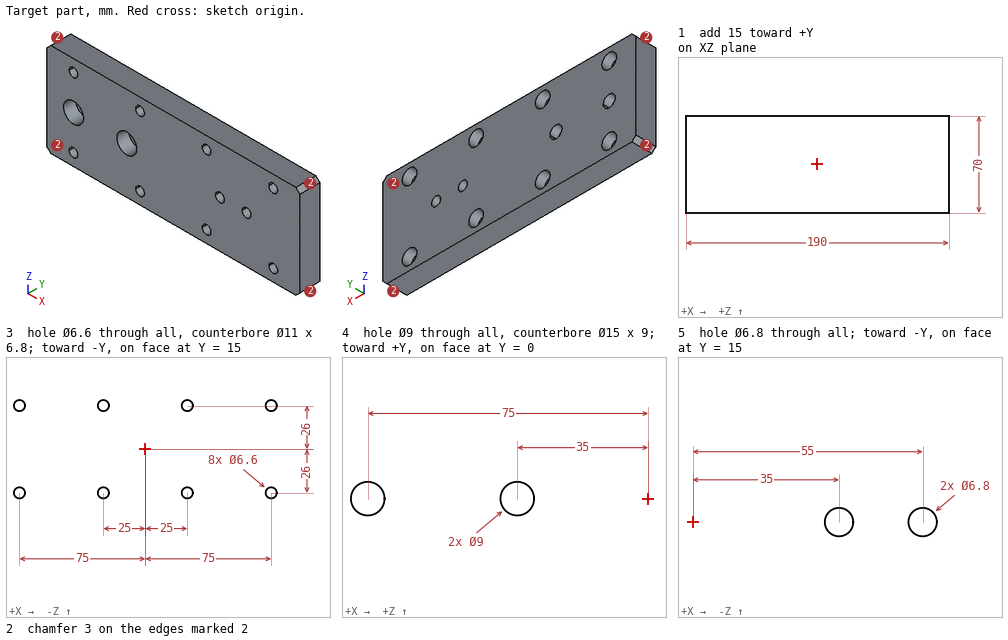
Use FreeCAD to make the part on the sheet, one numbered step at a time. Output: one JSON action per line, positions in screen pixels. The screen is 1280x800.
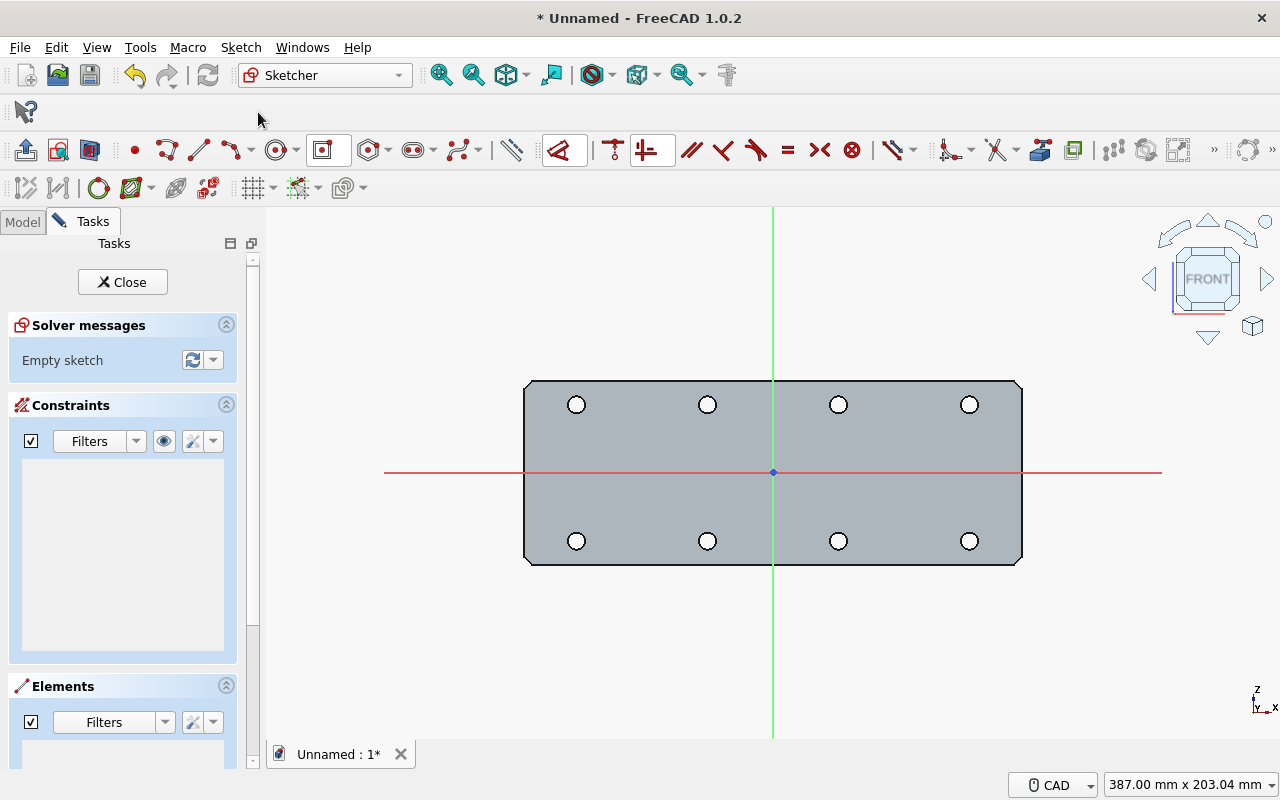
{"action": "scroll", "coordinate": [648, 473], "scroll_direction": "up", "scroll_amount": 5}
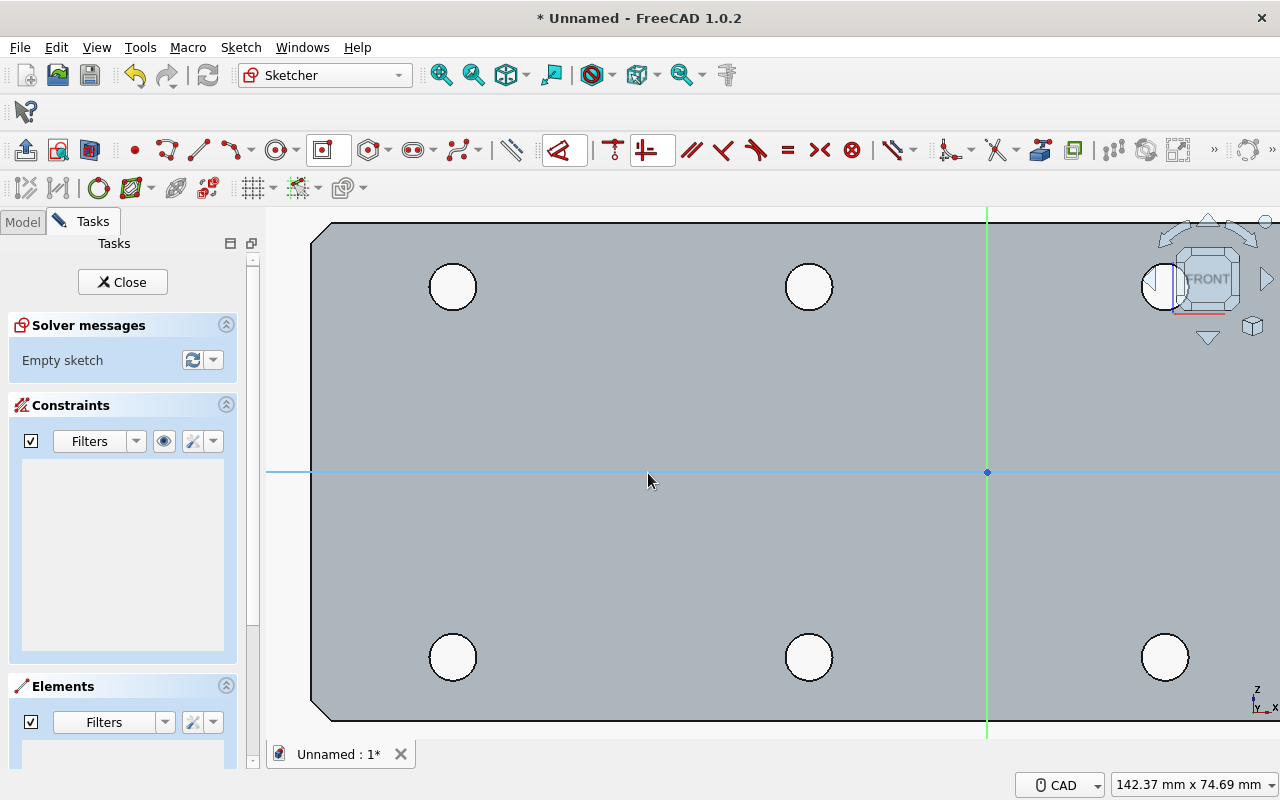
{"action": "left_click", "coordinate": [276, 150]}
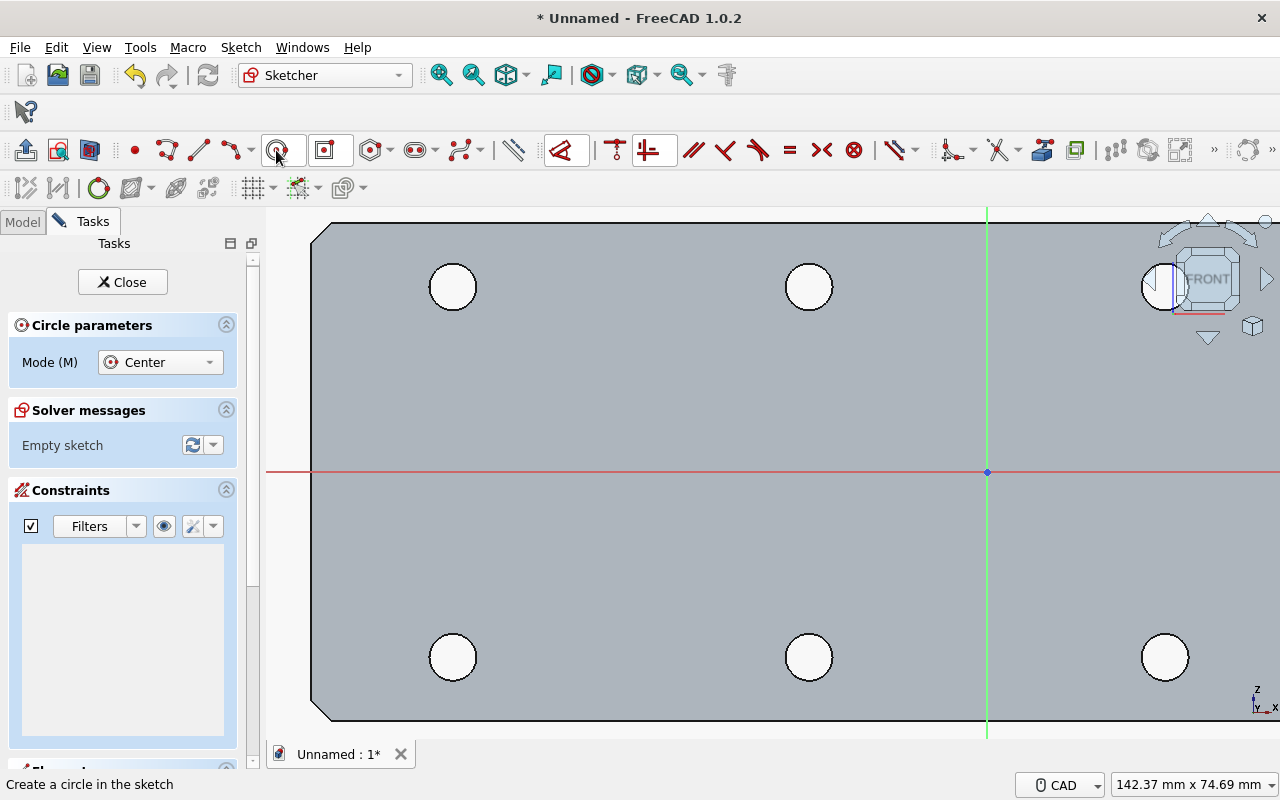
{"action": "left_click", "coordinate": [738, 472]}
{"action": "mouse_move", "coordinate": [761, 449]}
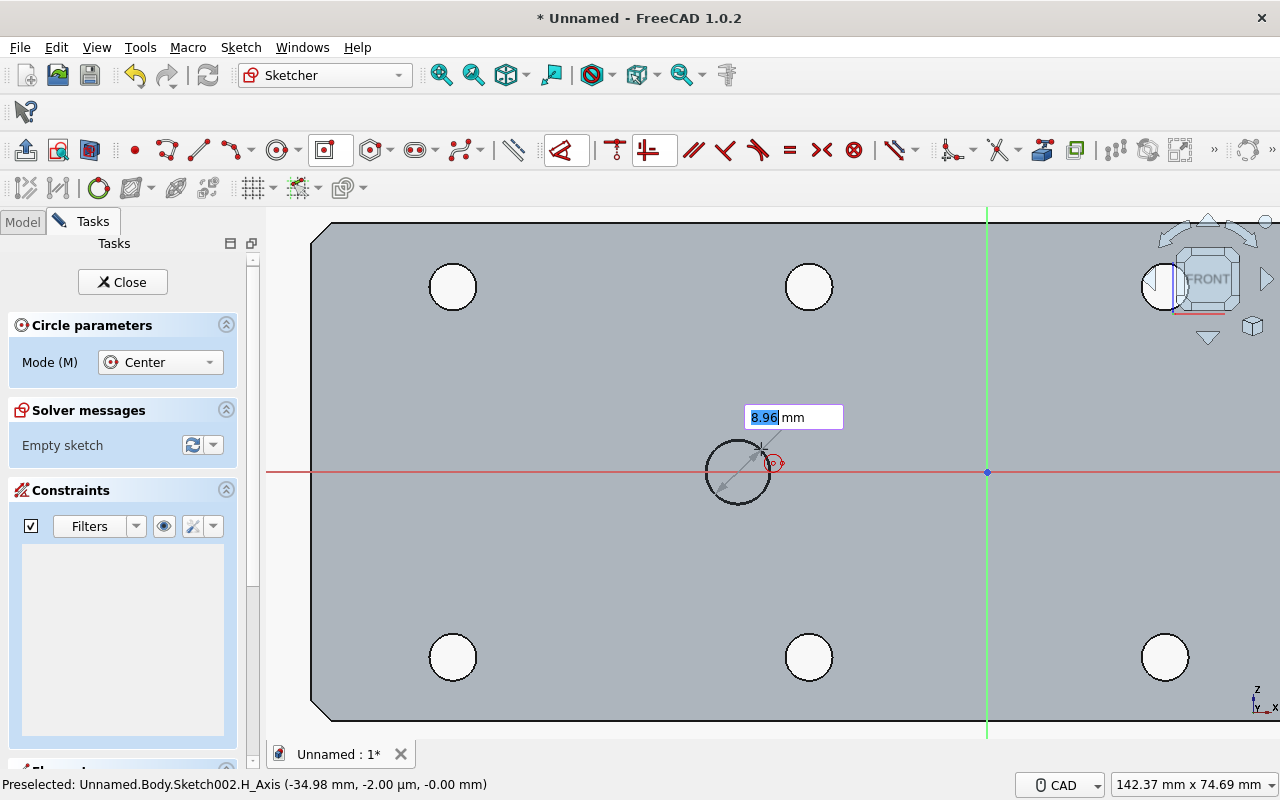
{"action": "type", "text": "9"}
{"action": "key", "text": "Return"}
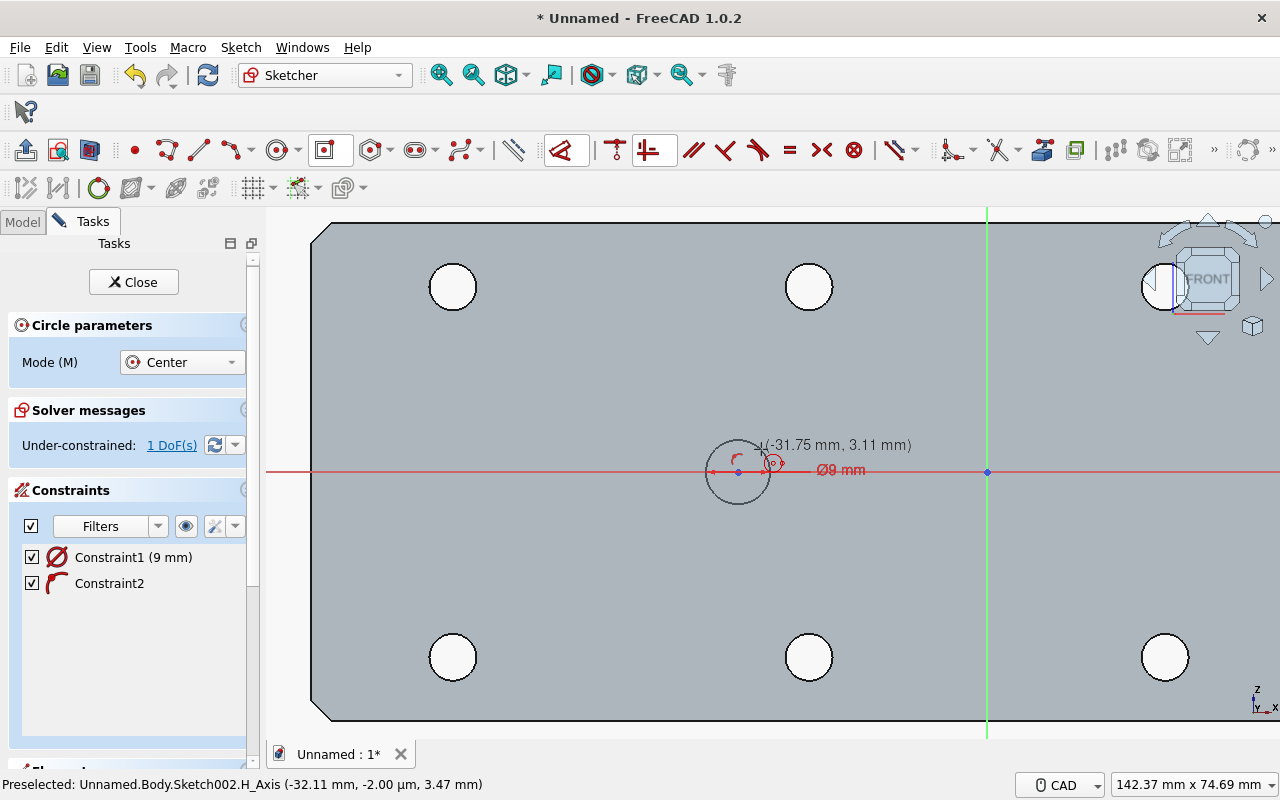
{"action": "left_click", "coordinate": [453, 472]}
{"action": "mouse_move", "coordinate": [476, 449]}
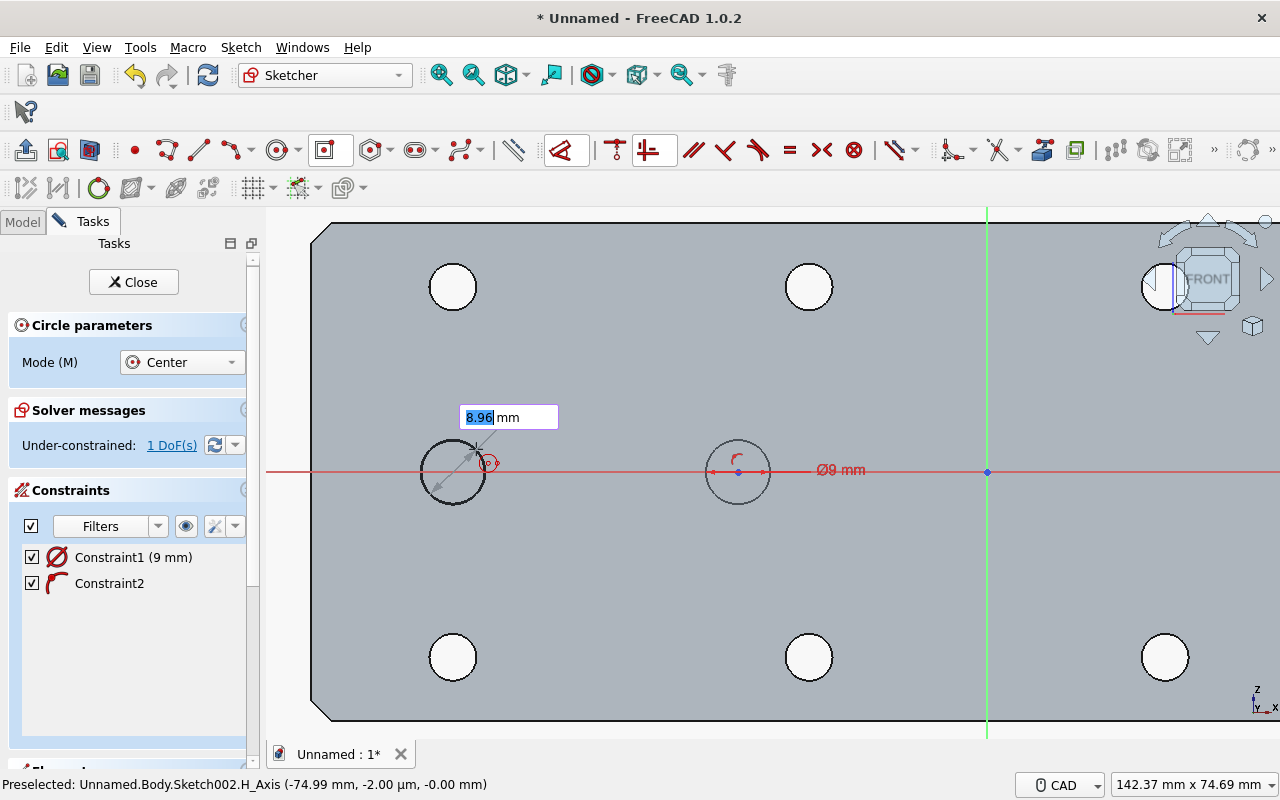
{"action": "type", "text": "9"}
{"action": "key", "text": "Return"}
{"action": "key", "text": "Escape"}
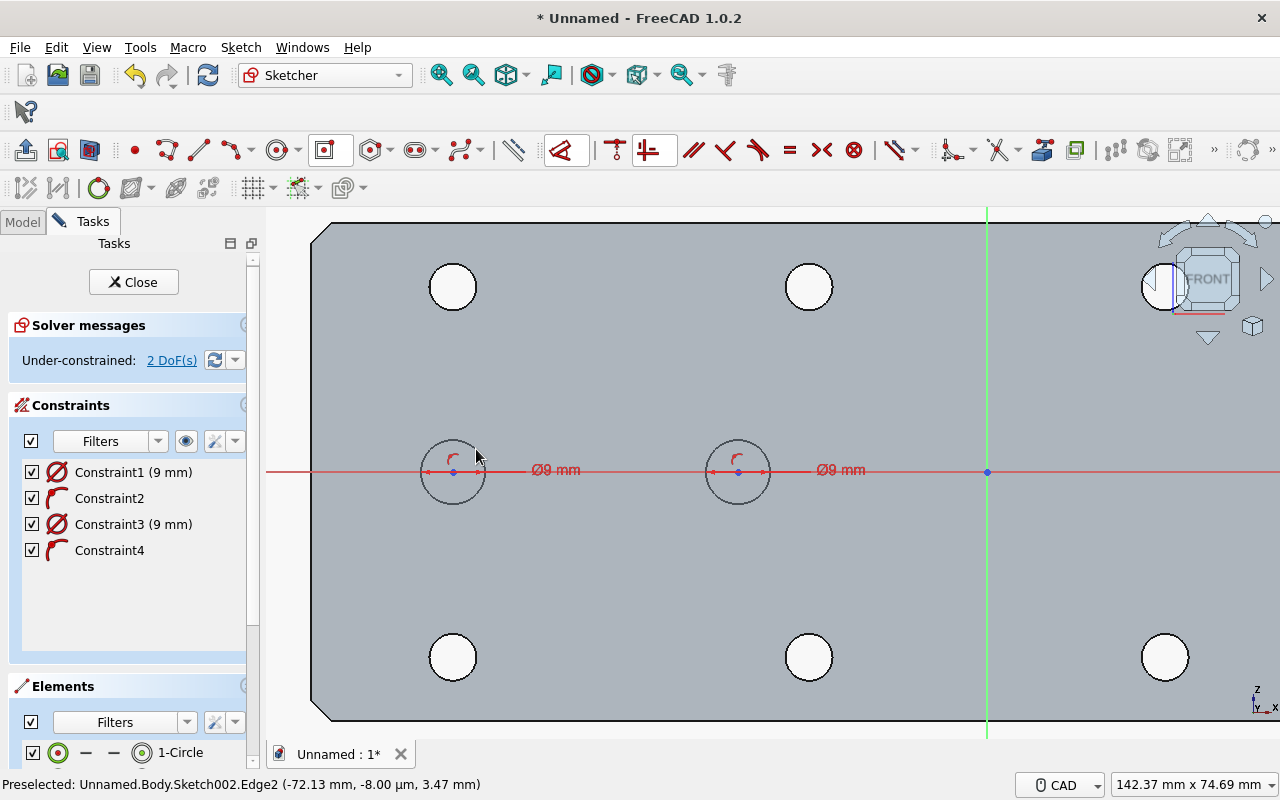
{"action": "key", "text": "d"}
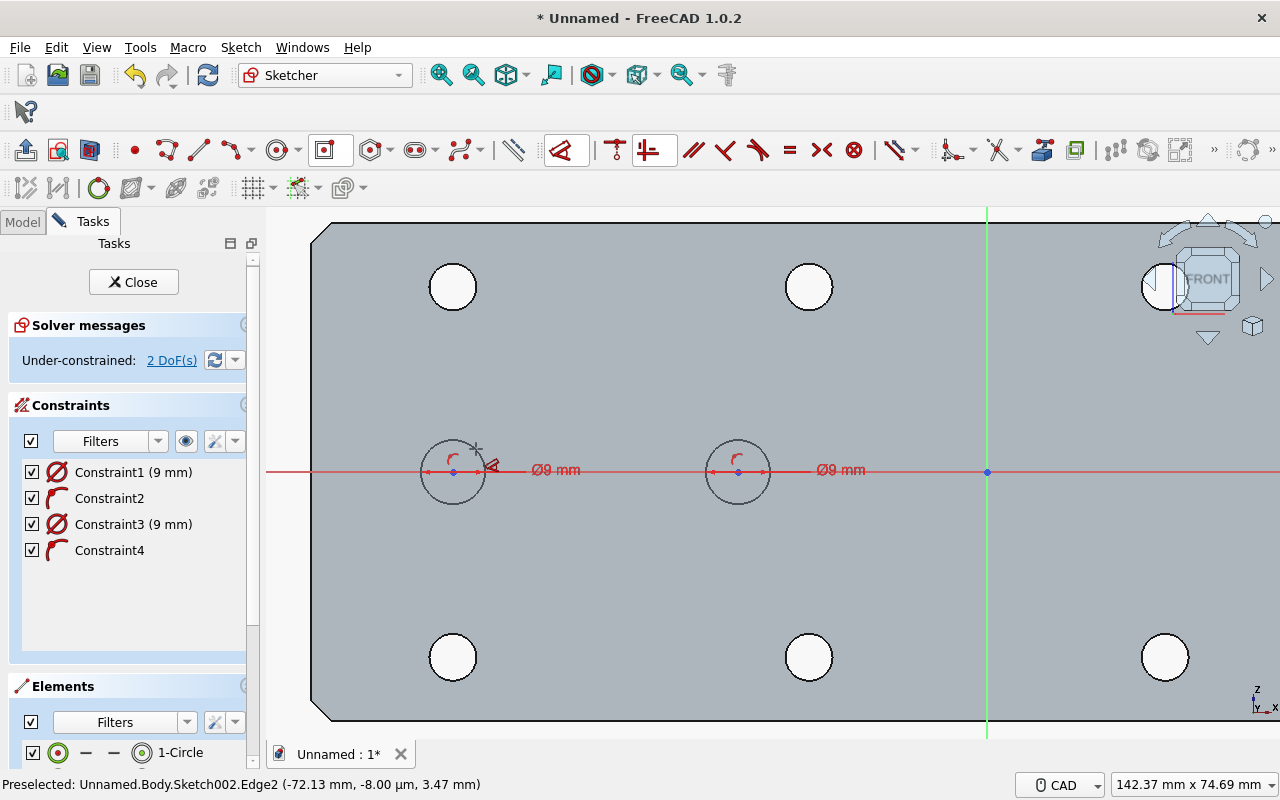
{"action": "left_click", "coordinate": [738, 472]}
{"action": "left_click", "coordinate": [863, 506]}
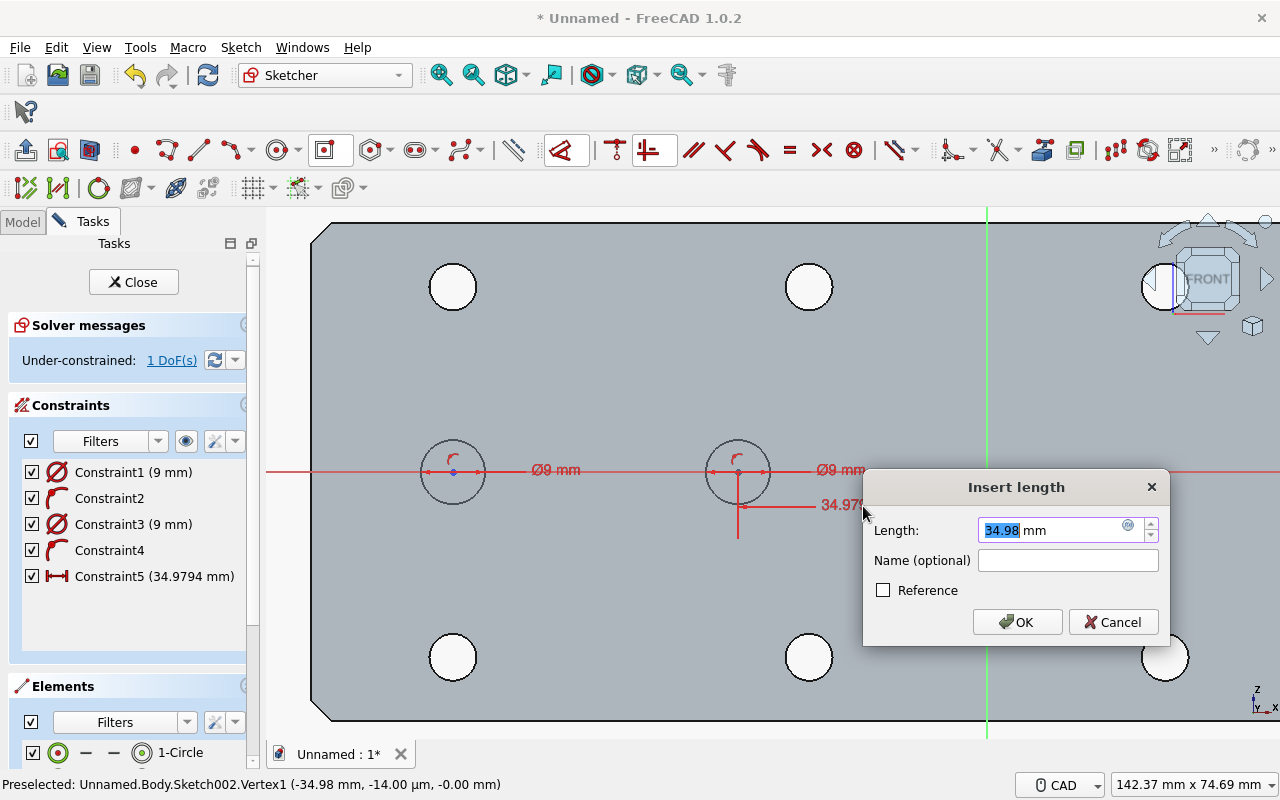
{"action": "type", "text": "35"}
{"action": "key", "text": "Return"}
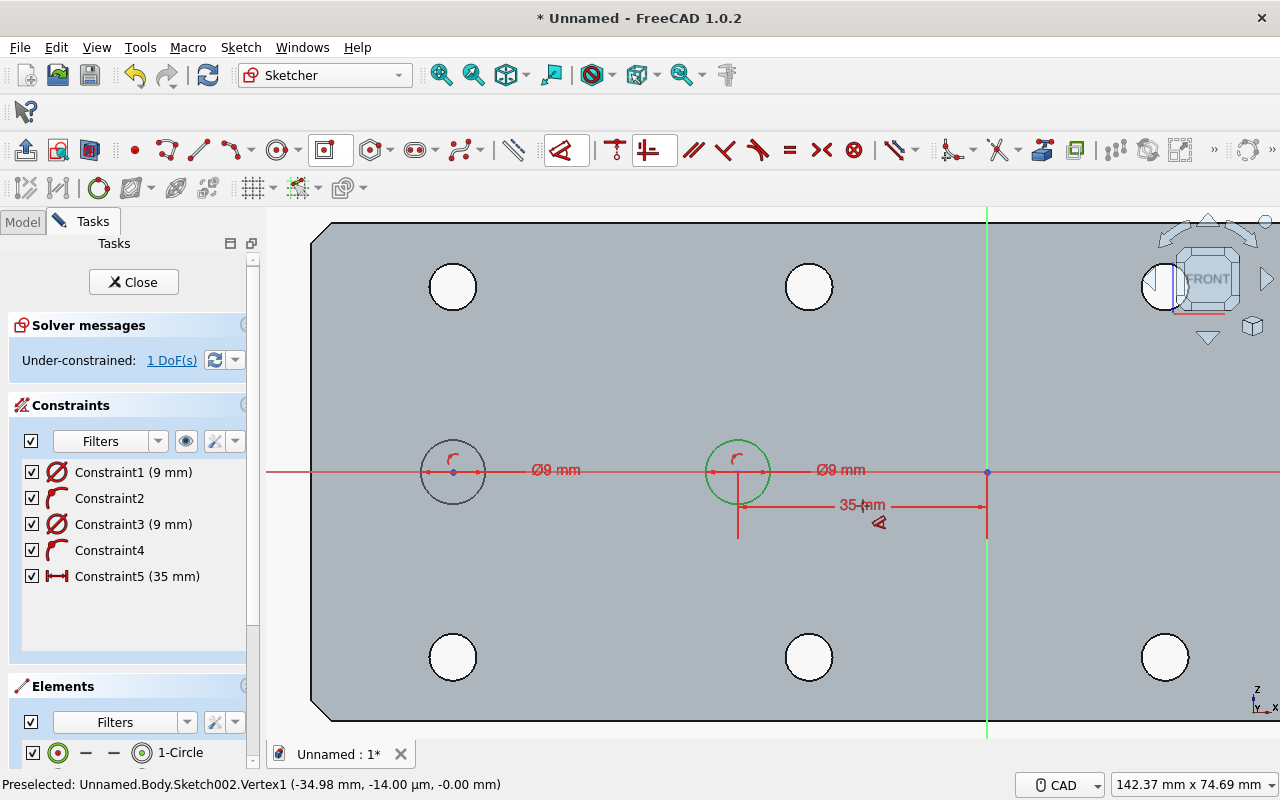
{"action": "left_click", "coordinate": [453, 472]}
{"action": "left_click", "coordinate": [597, 506]}